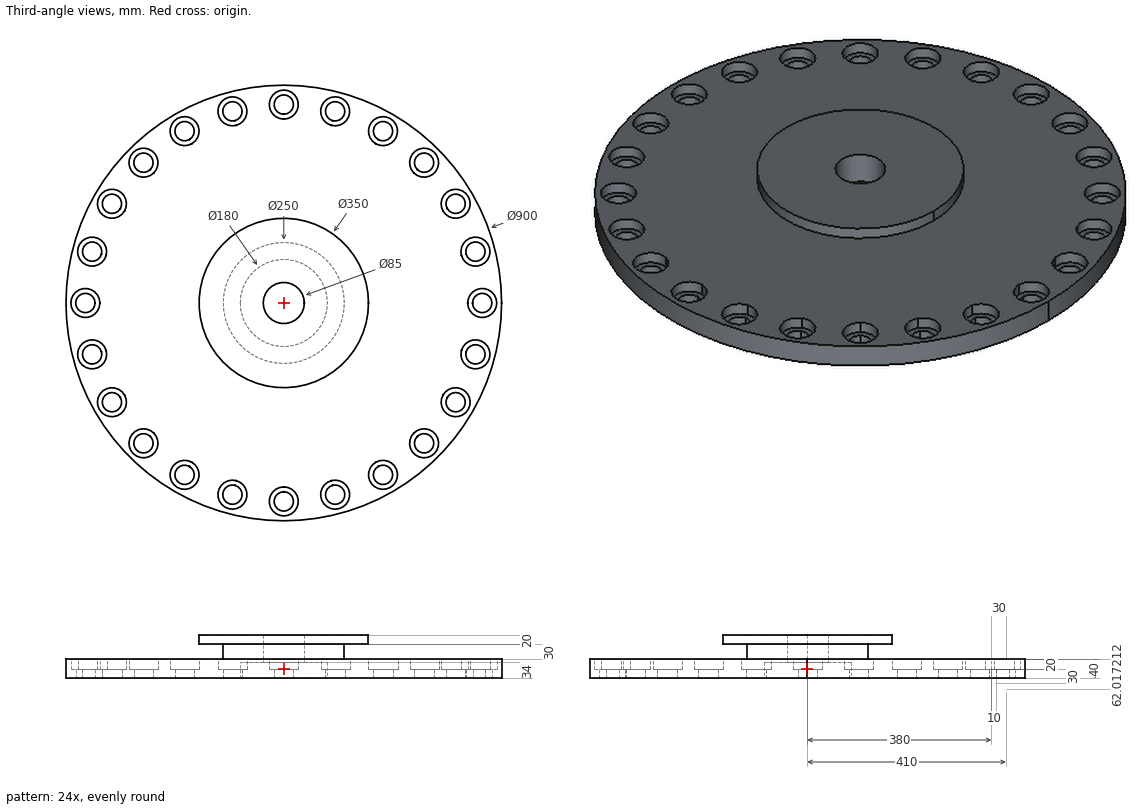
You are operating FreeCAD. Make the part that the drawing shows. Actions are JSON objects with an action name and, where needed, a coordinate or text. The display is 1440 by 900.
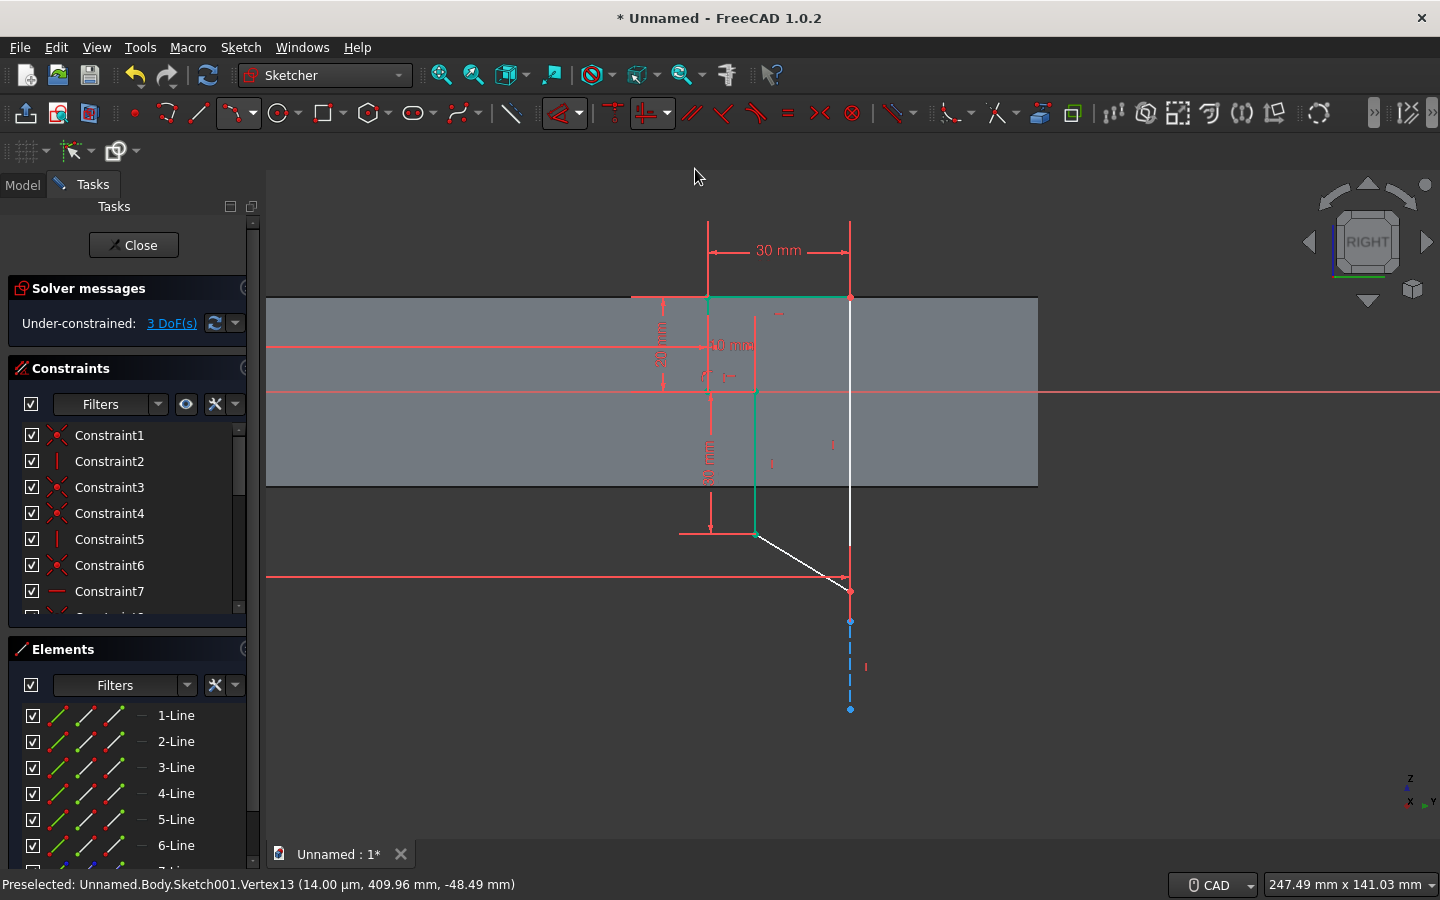
{"action": "left_click", "coordinate": [850, 504]}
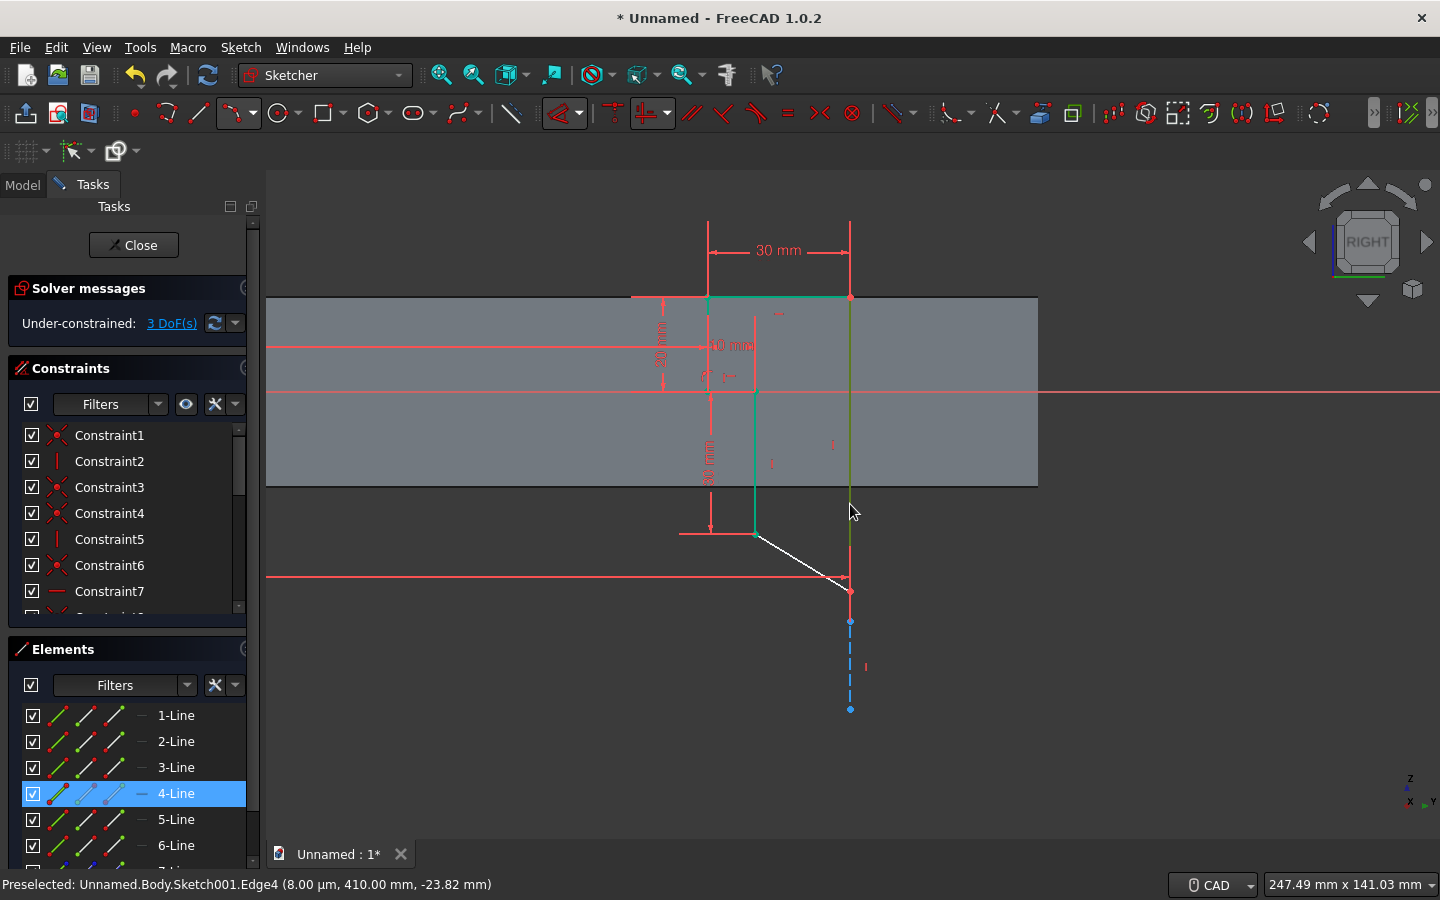
{"action": "left_click", "coordinate": [582, 114]}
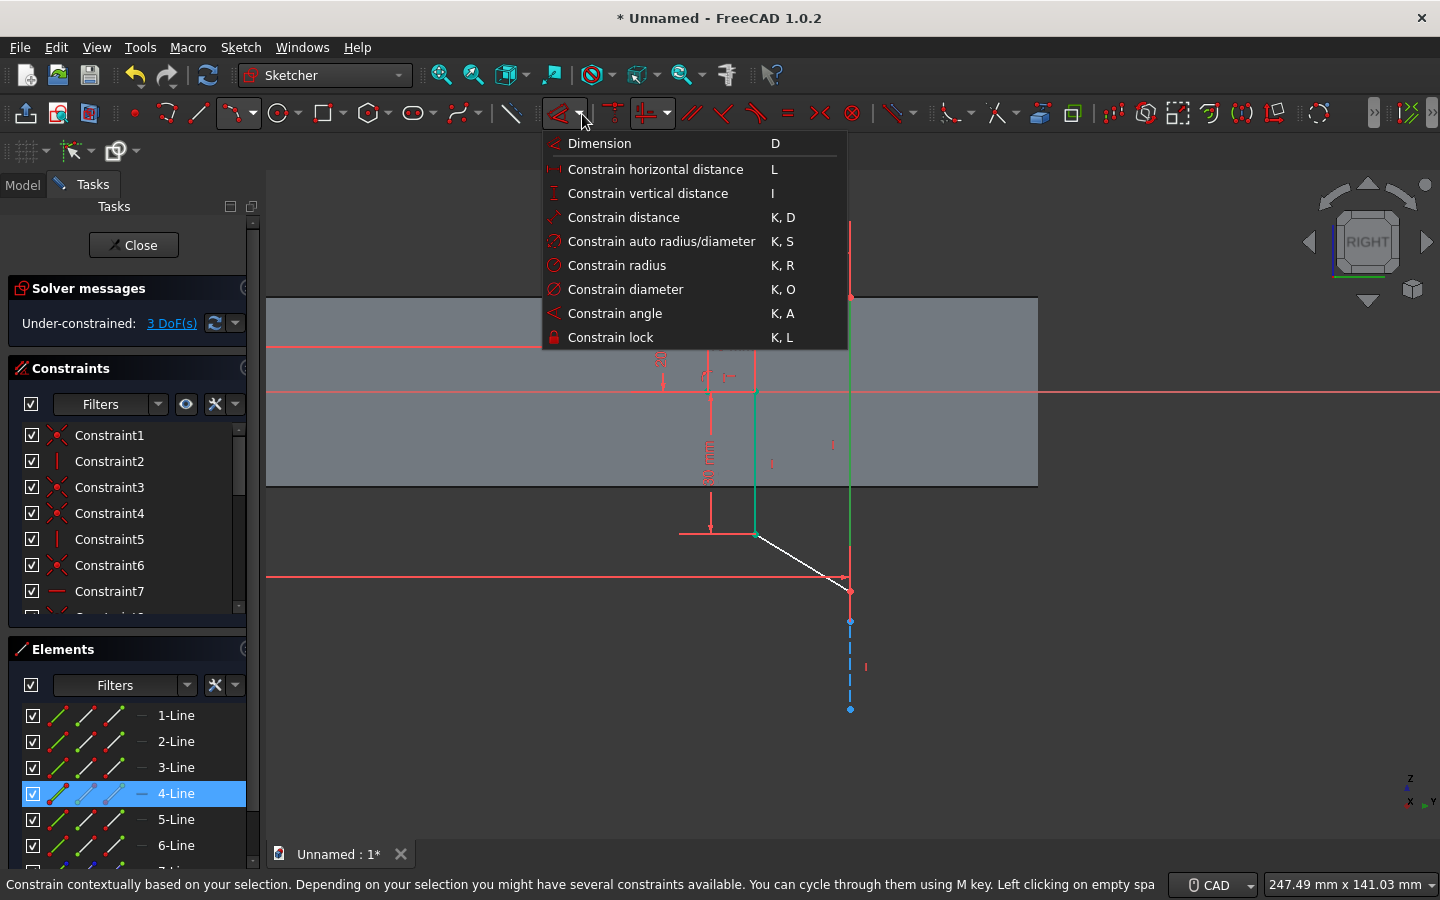
{"action": "left_click", "coordinate": [695, 193]}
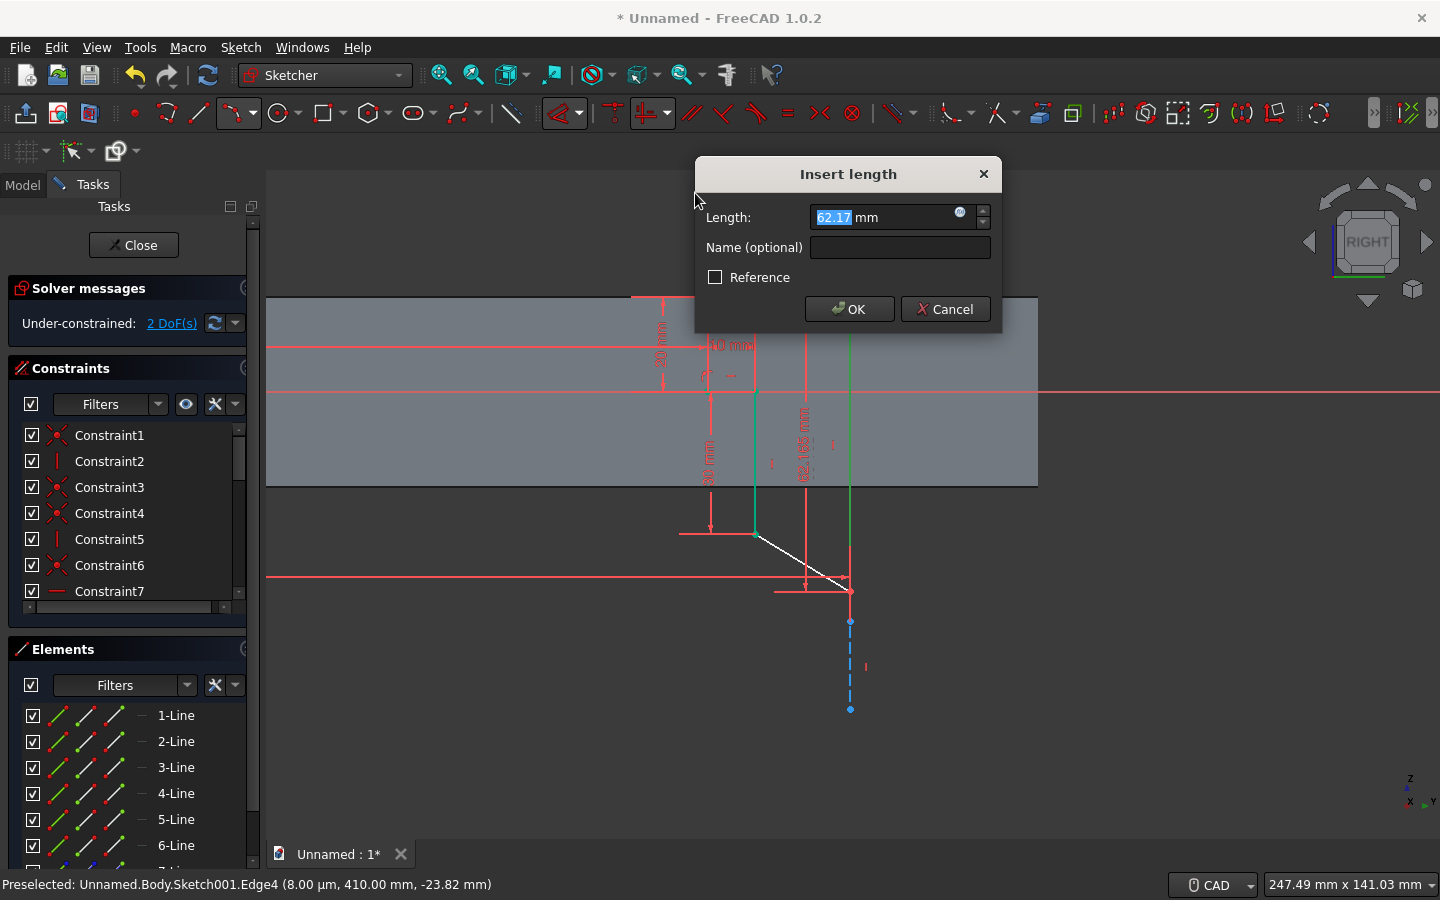
{"action": "type", "text": "62.017212"}
{"action": "key", "text": "Return"}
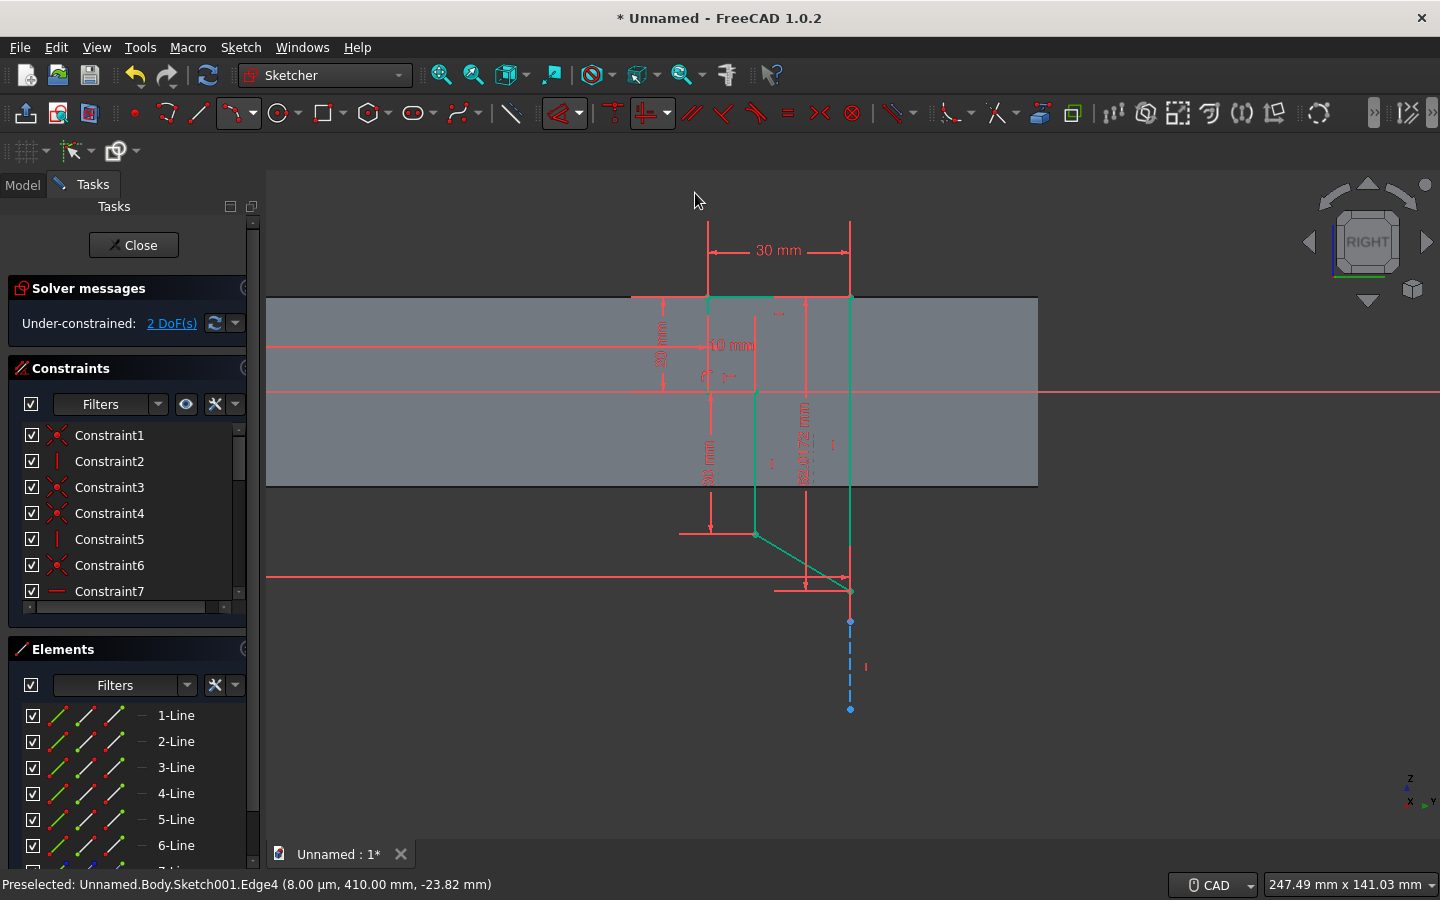
{"action": "left_click", "coordinate": [134, 245]}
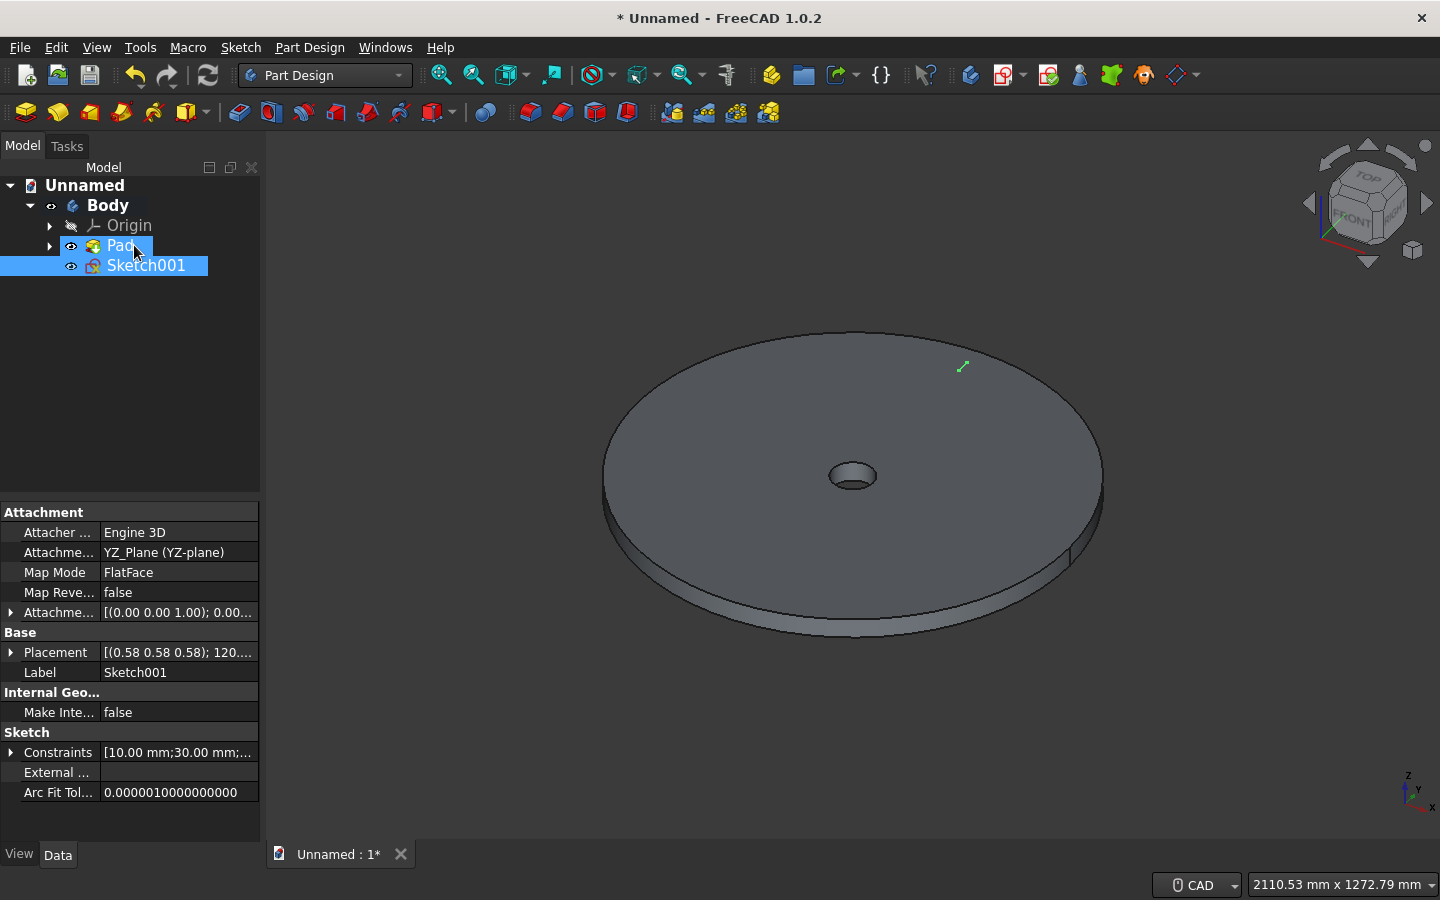
{"action": "left_click", "coordinate": [304, 112]}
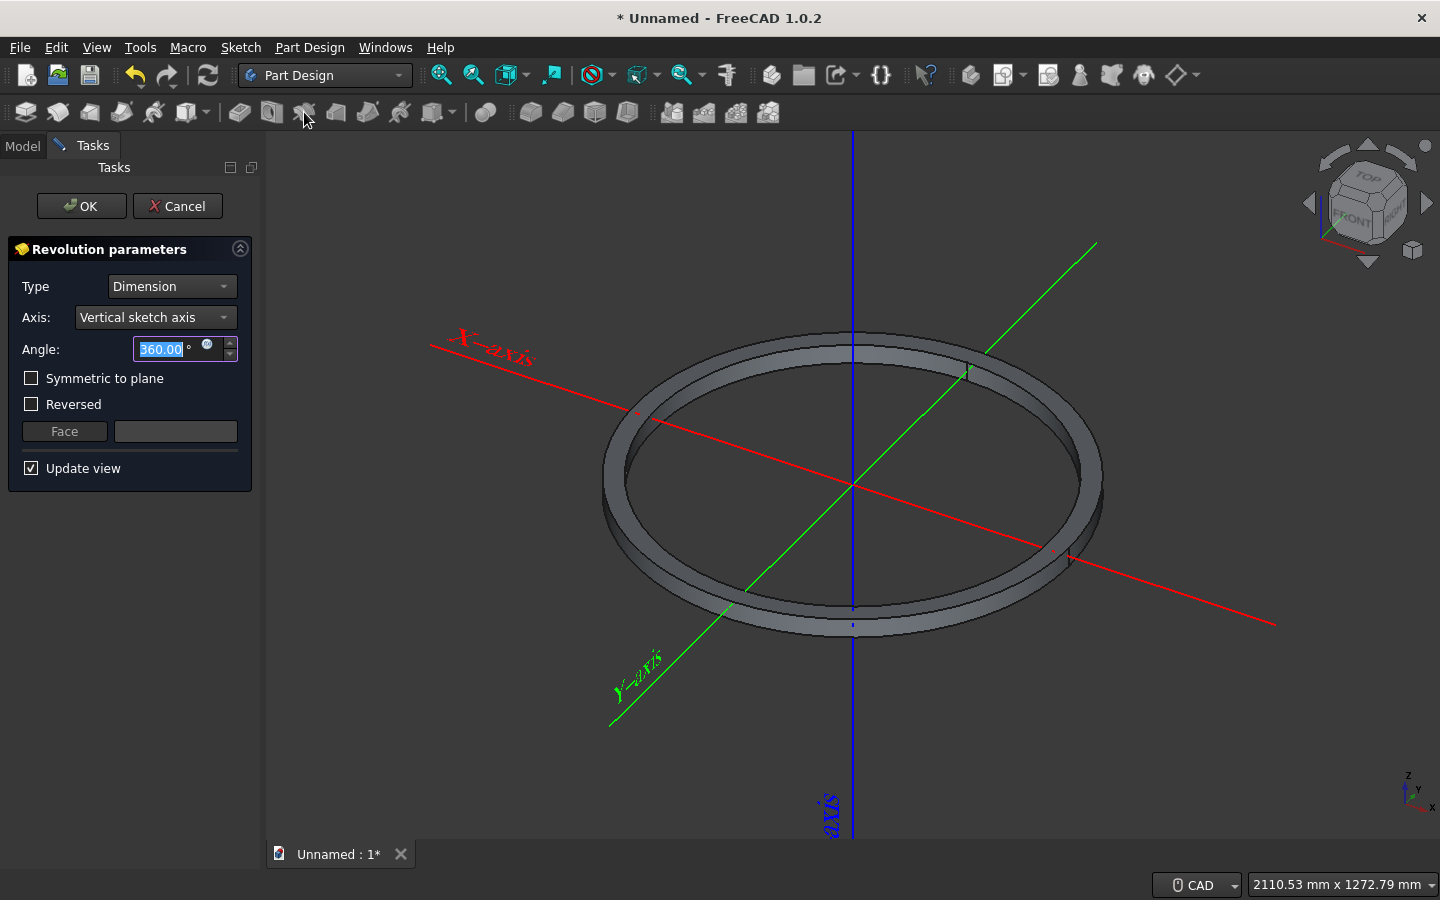
{"action": "left_click", "coordinate": [156, 318]}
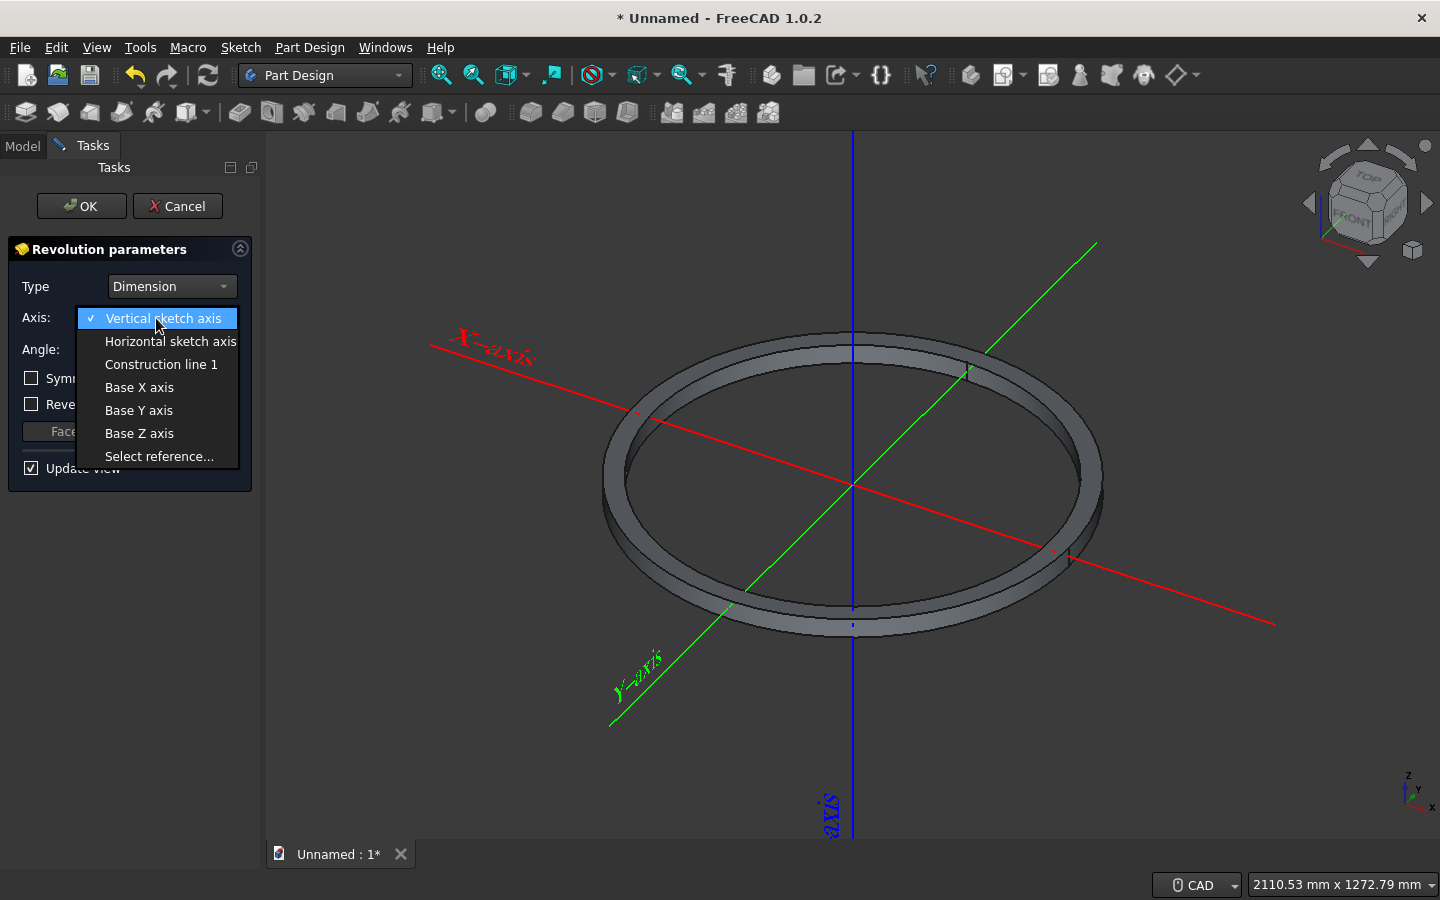
{"action": "left_click", "coordinate": [156, 364]}